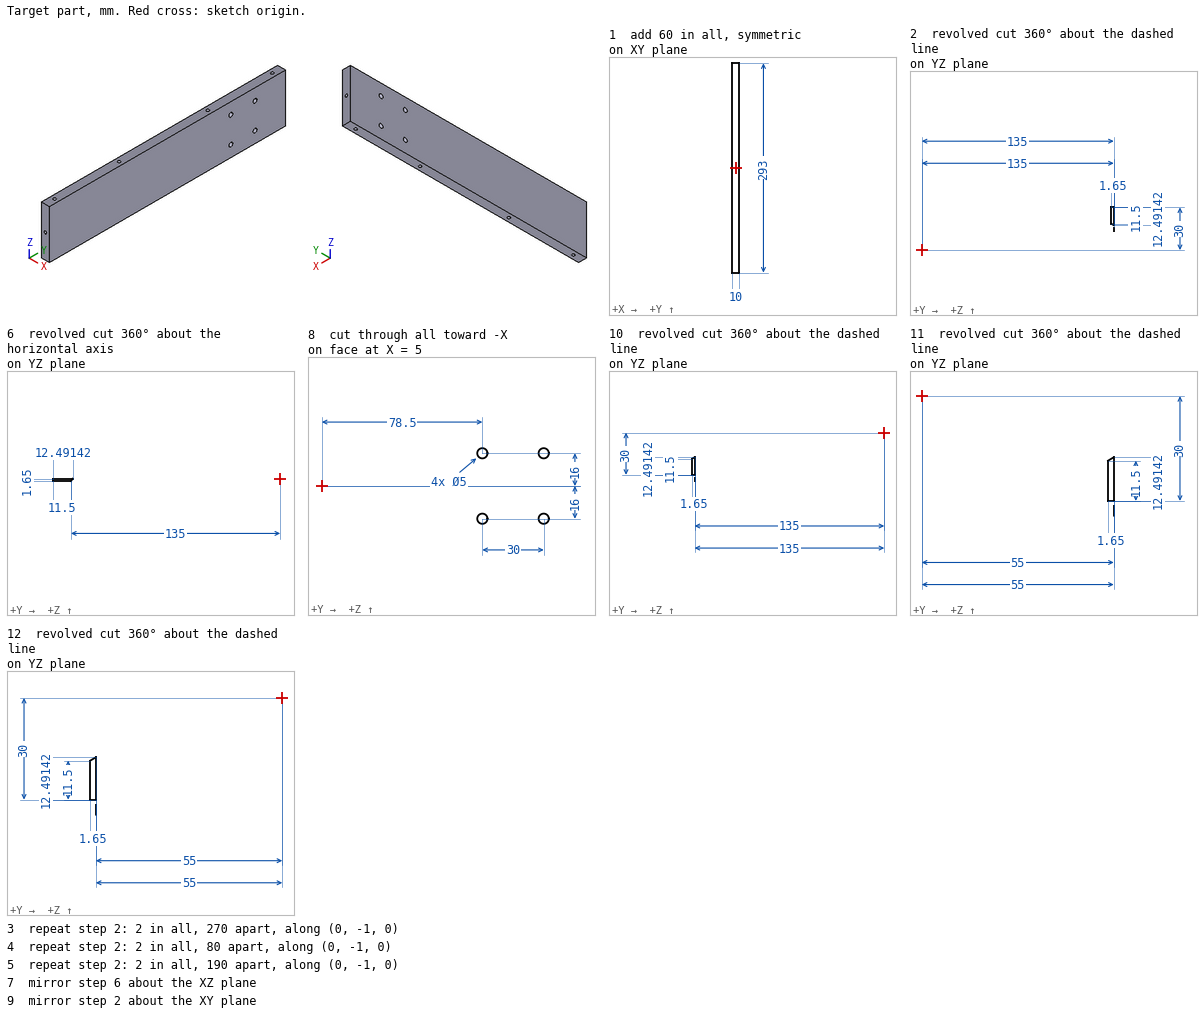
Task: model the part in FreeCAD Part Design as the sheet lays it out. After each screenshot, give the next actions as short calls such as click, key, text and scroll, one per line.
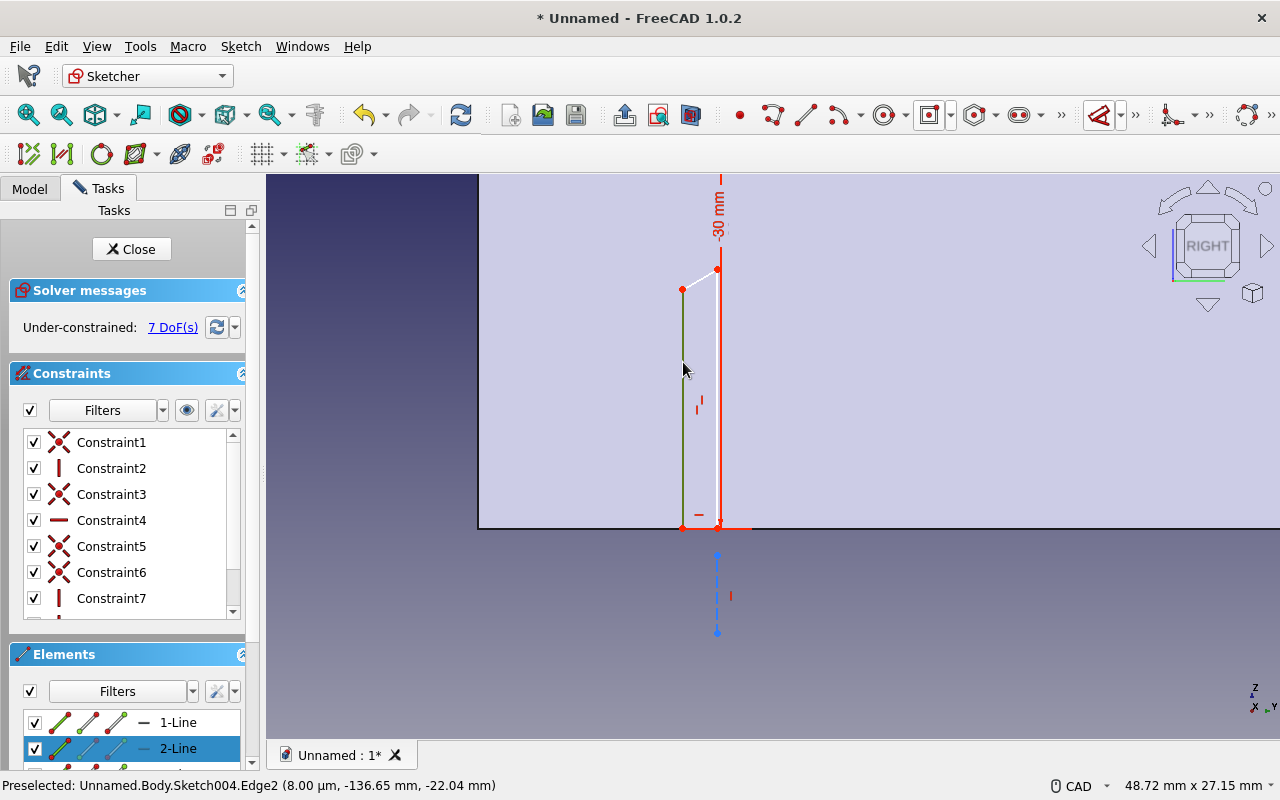
key(i)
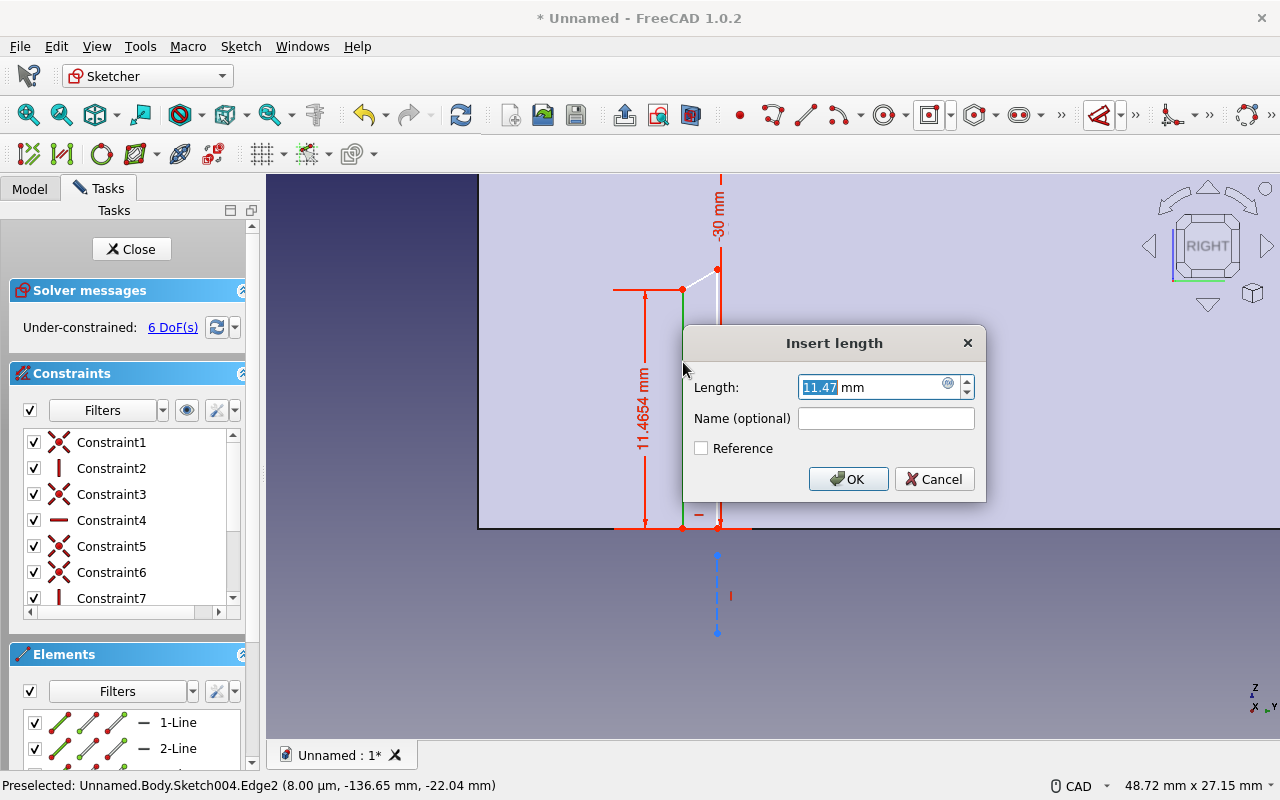
text(11.5)
key(Return)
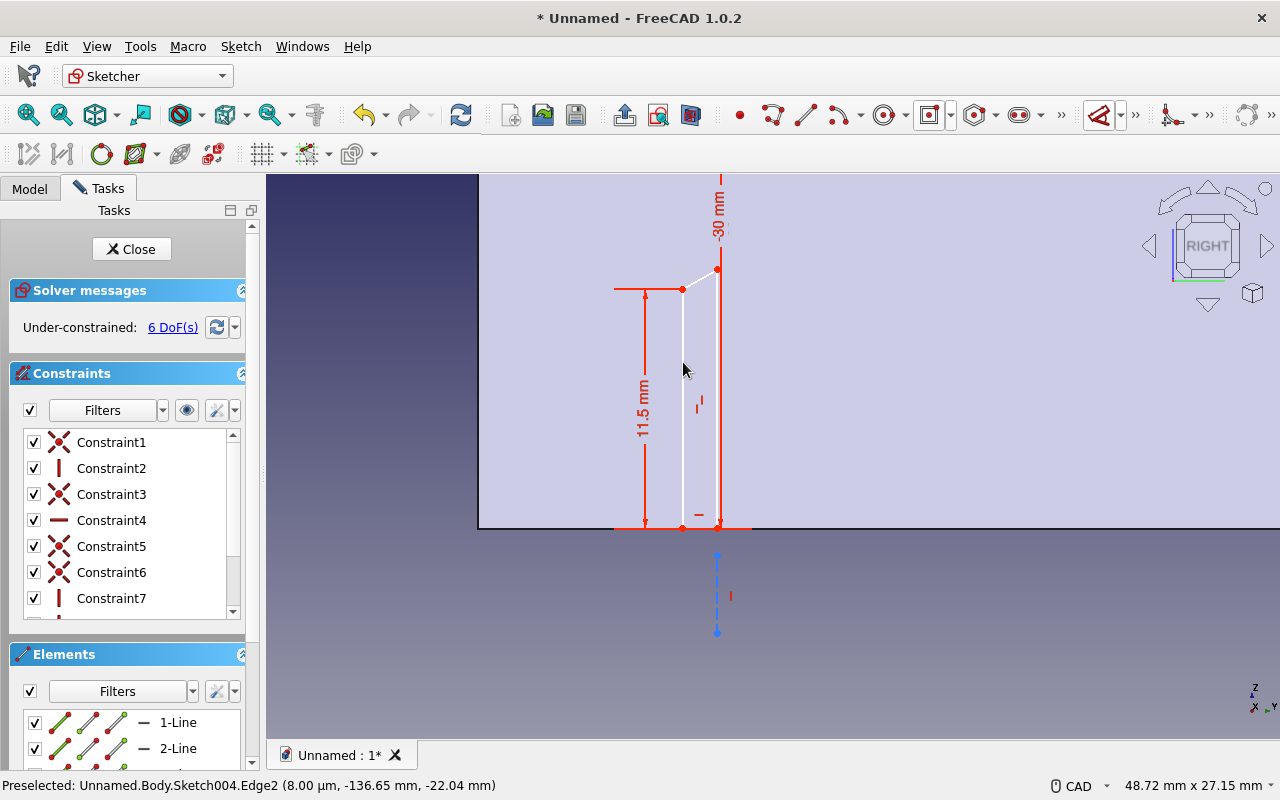
scroll(693, 529, up, 2)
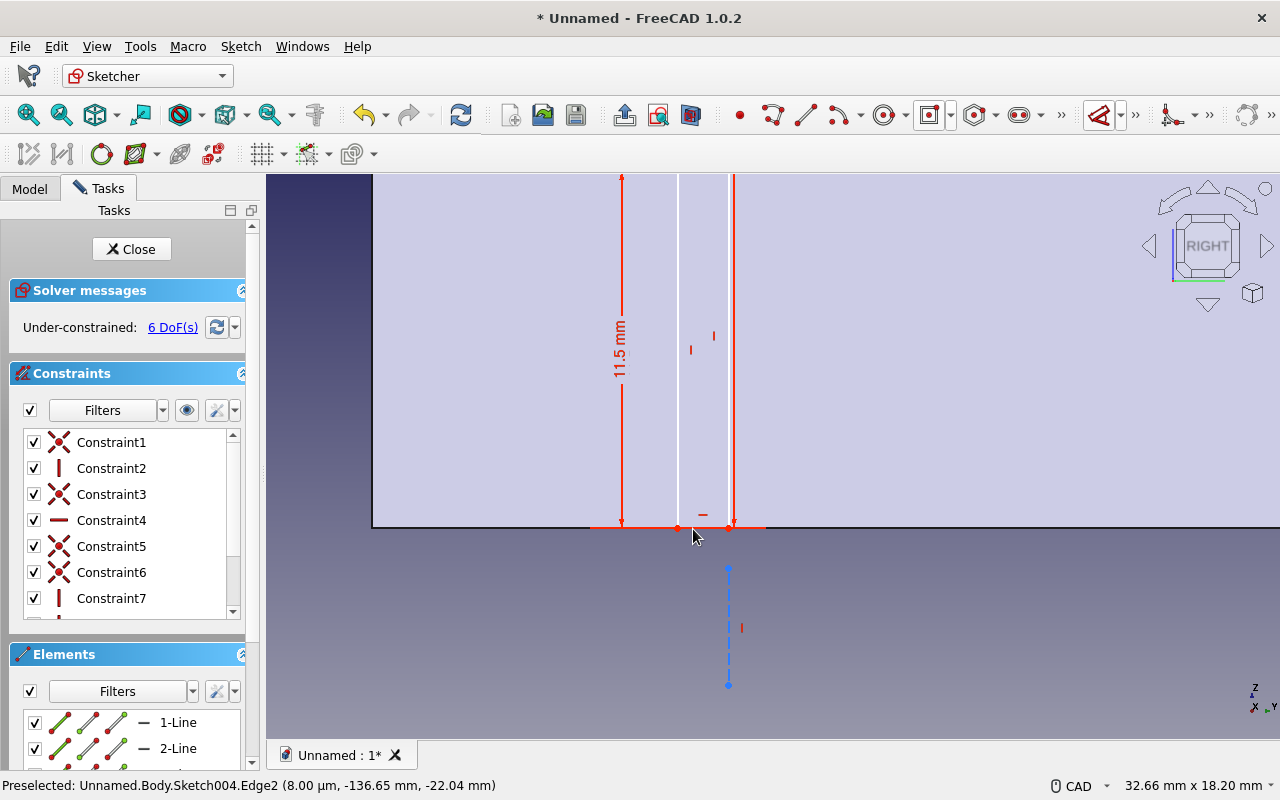
click(693, 528)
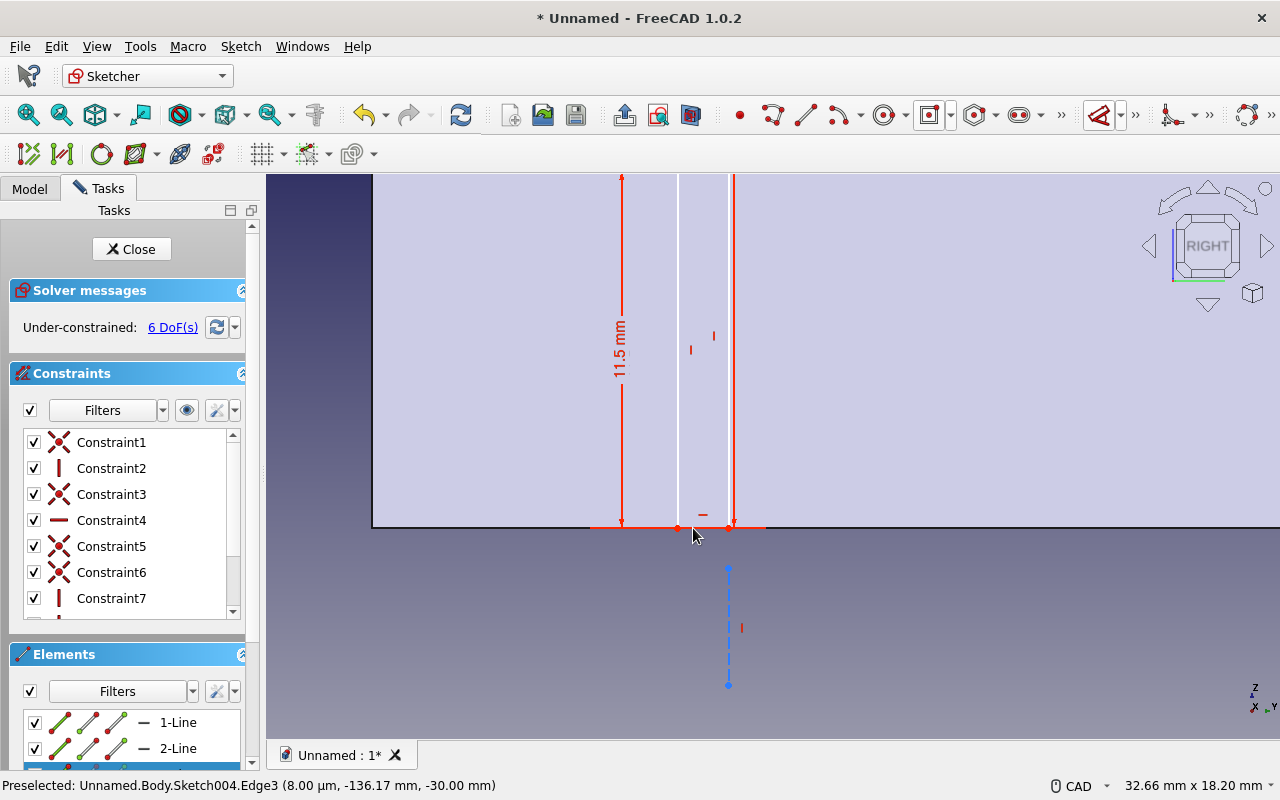
click(1120, 116)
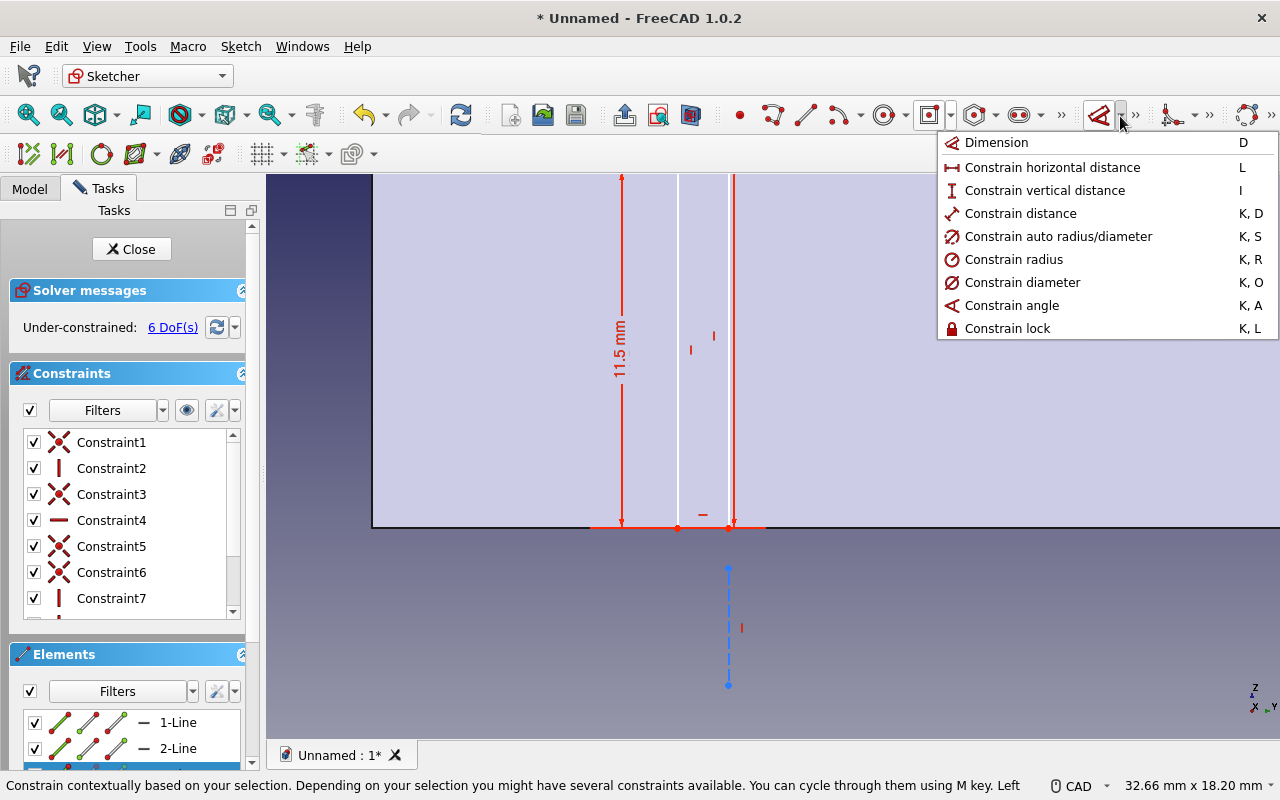
click(1108, 168)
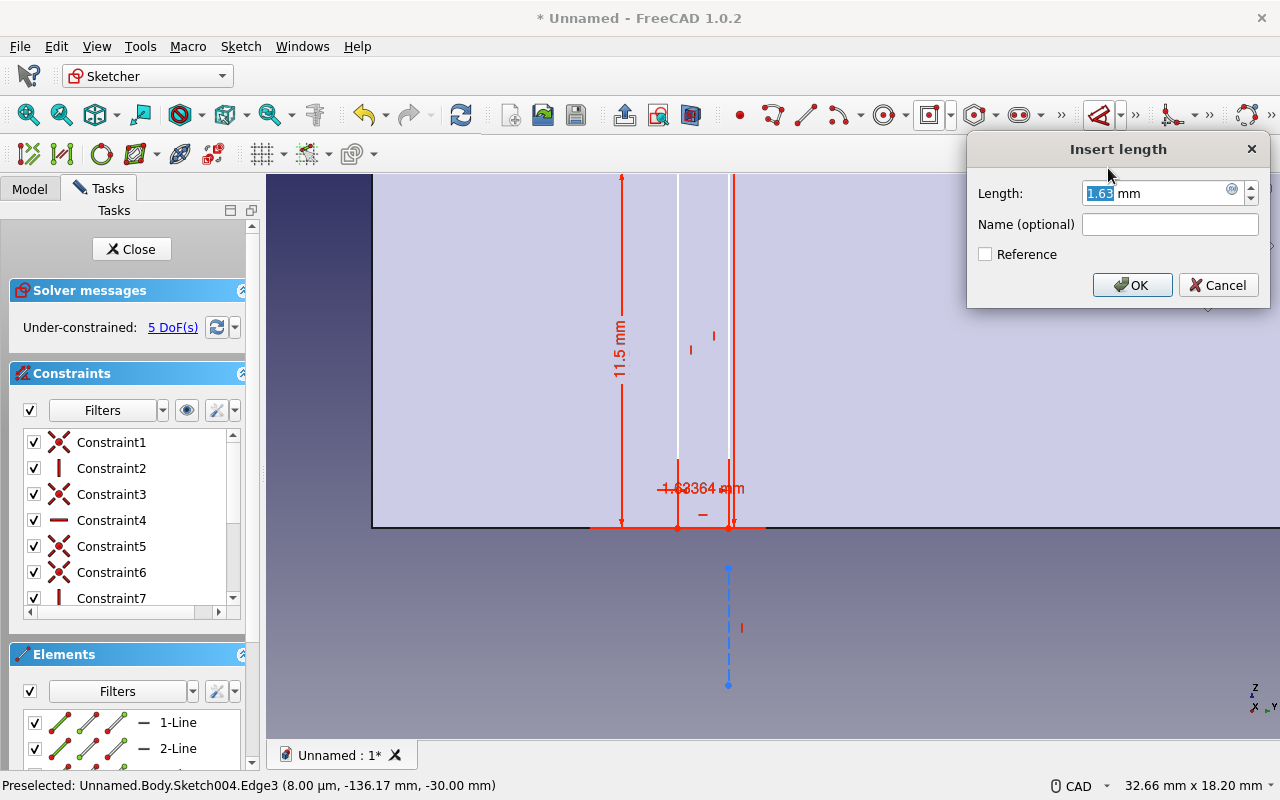
text(1.65)
key(Return)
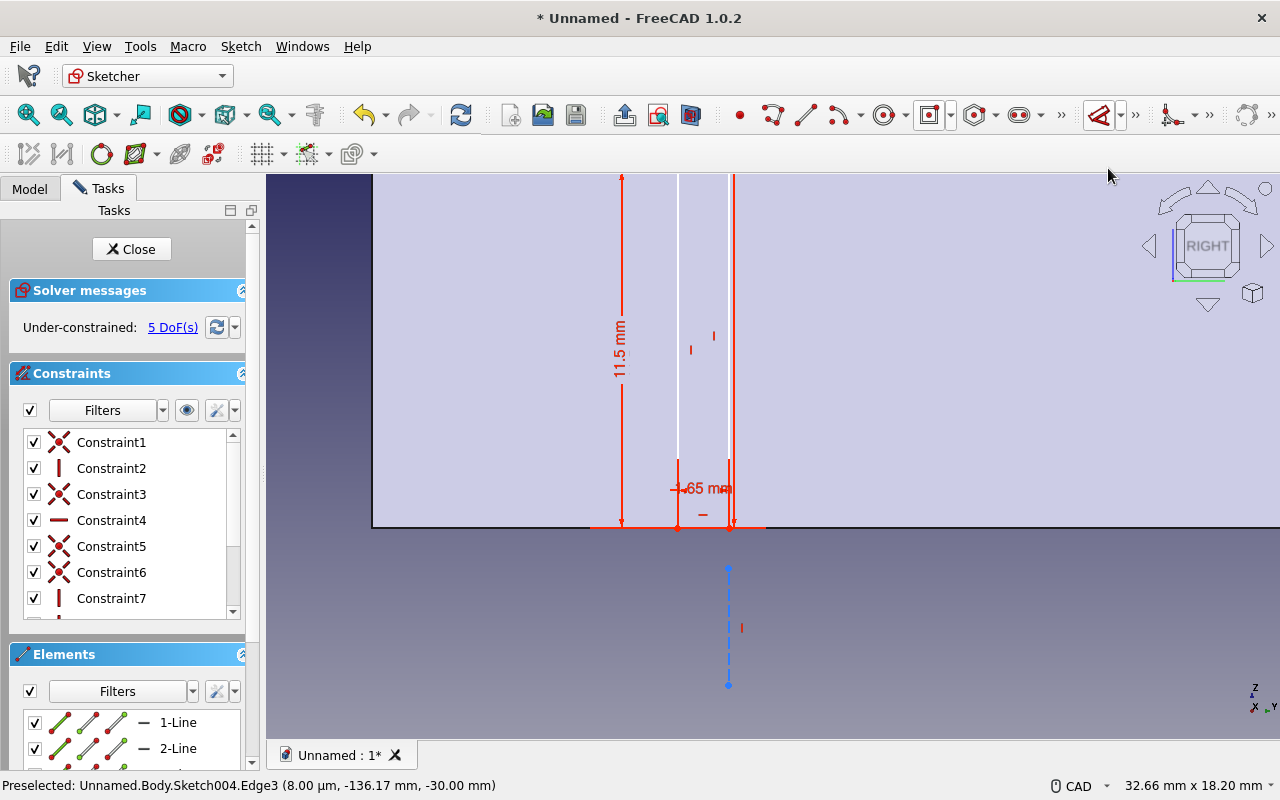
scroll(706, 547, down, 2)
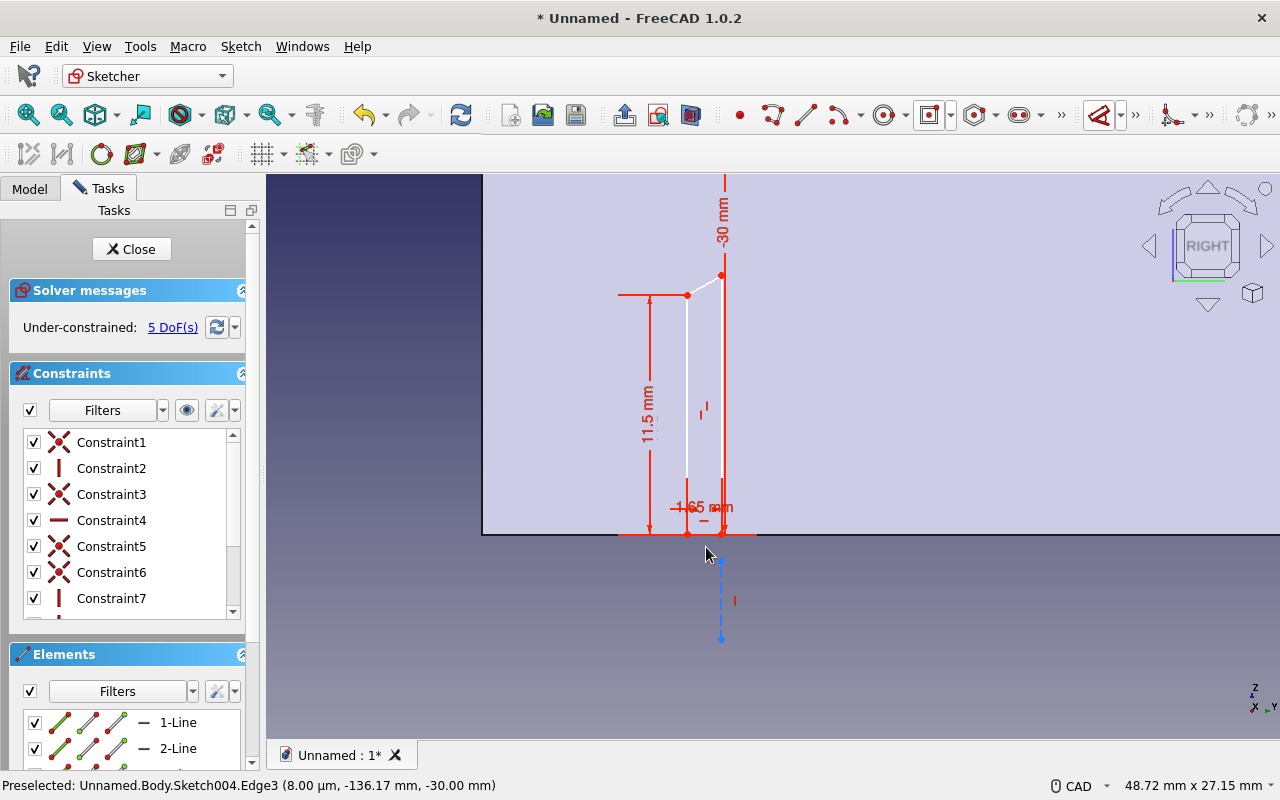
click(722, 276)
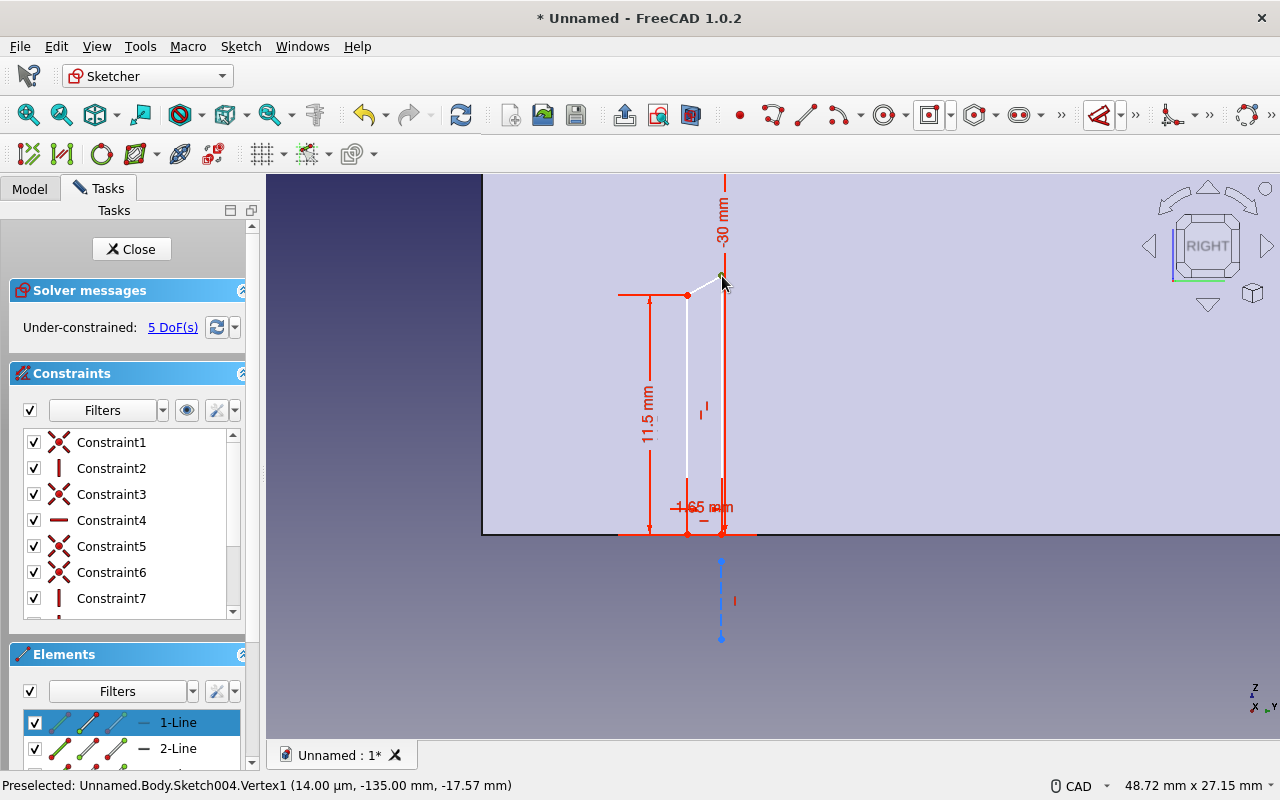
key(l)